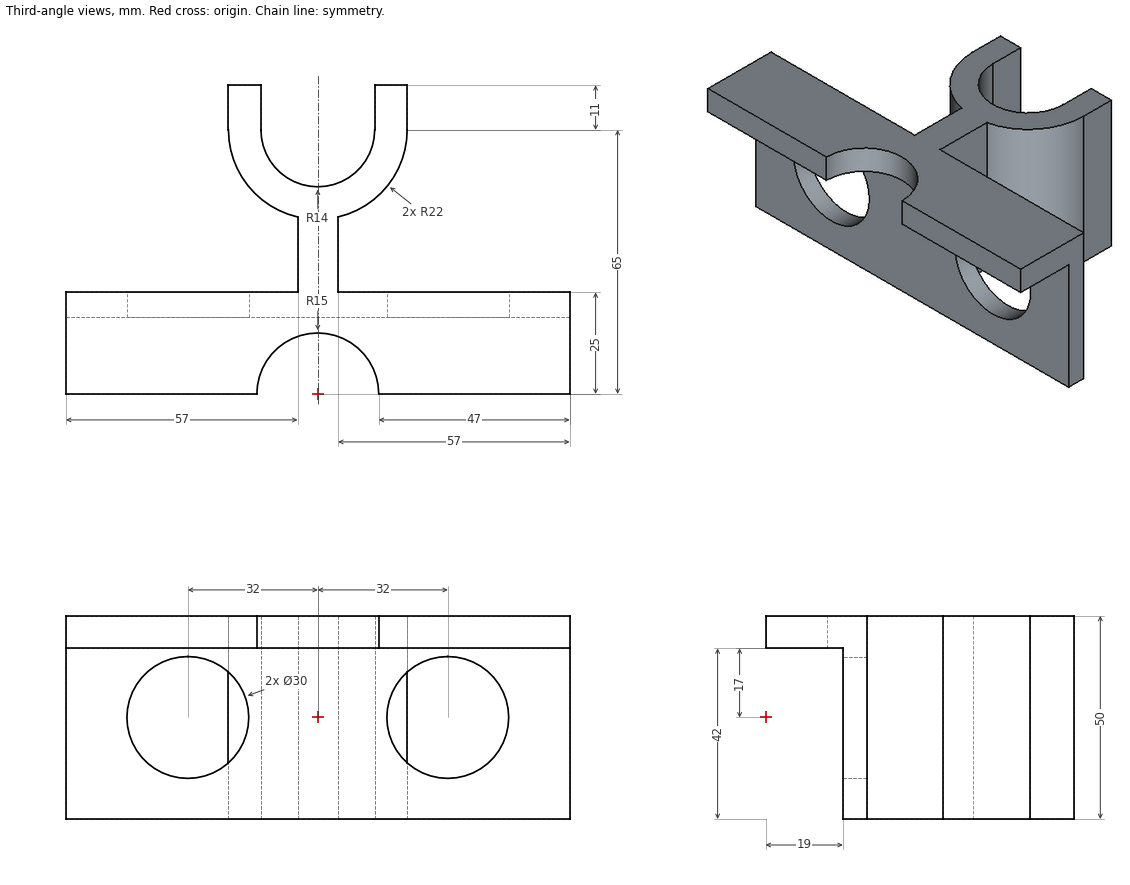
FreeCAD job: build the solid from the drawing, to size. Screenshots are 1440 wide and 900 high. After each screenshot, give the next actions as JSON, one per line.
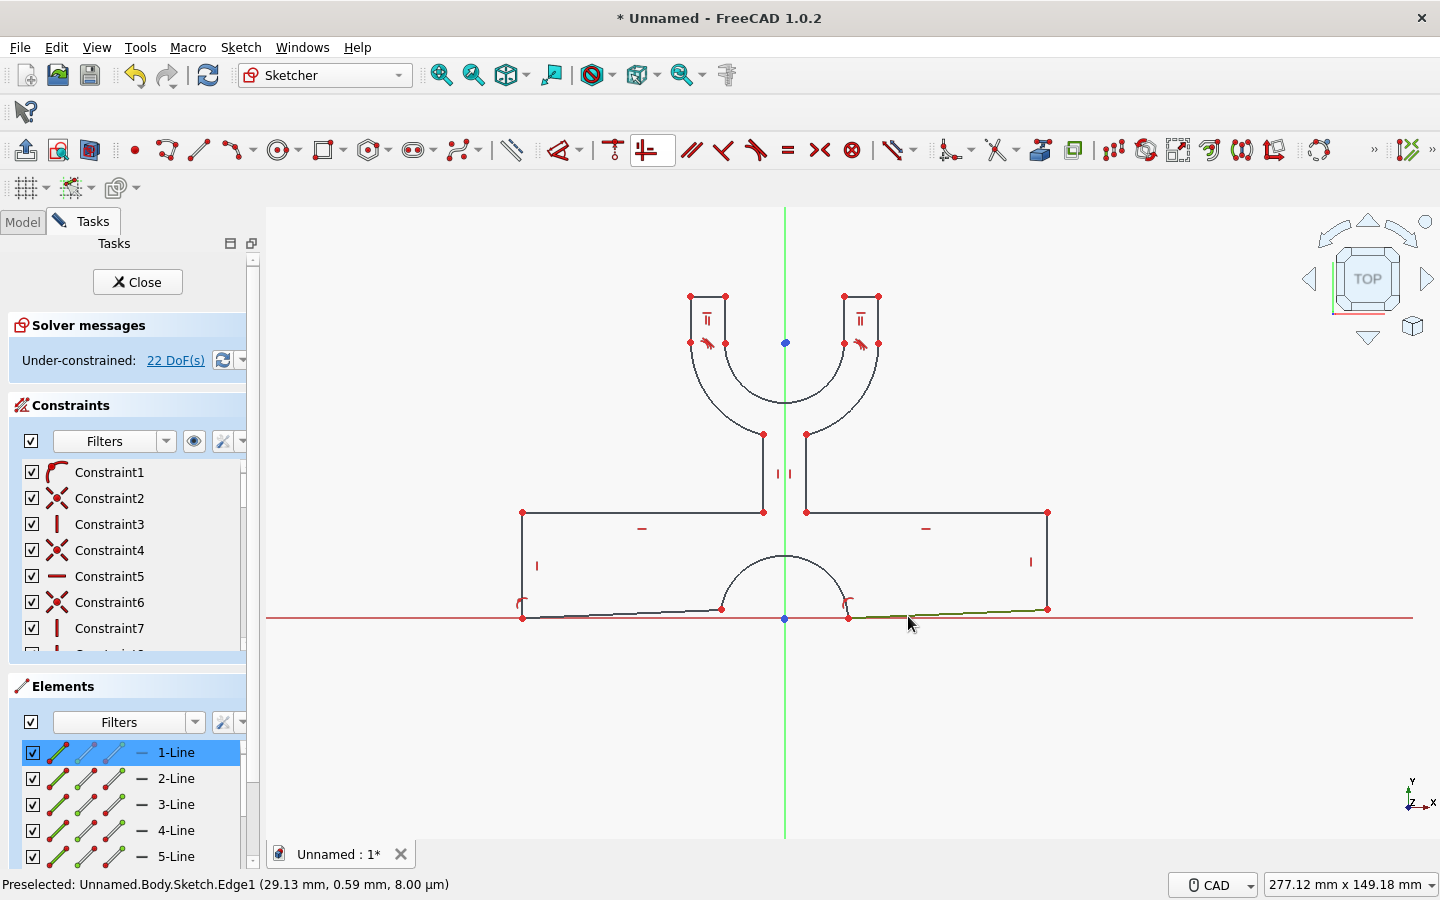
{"action": "key", "text": "h"}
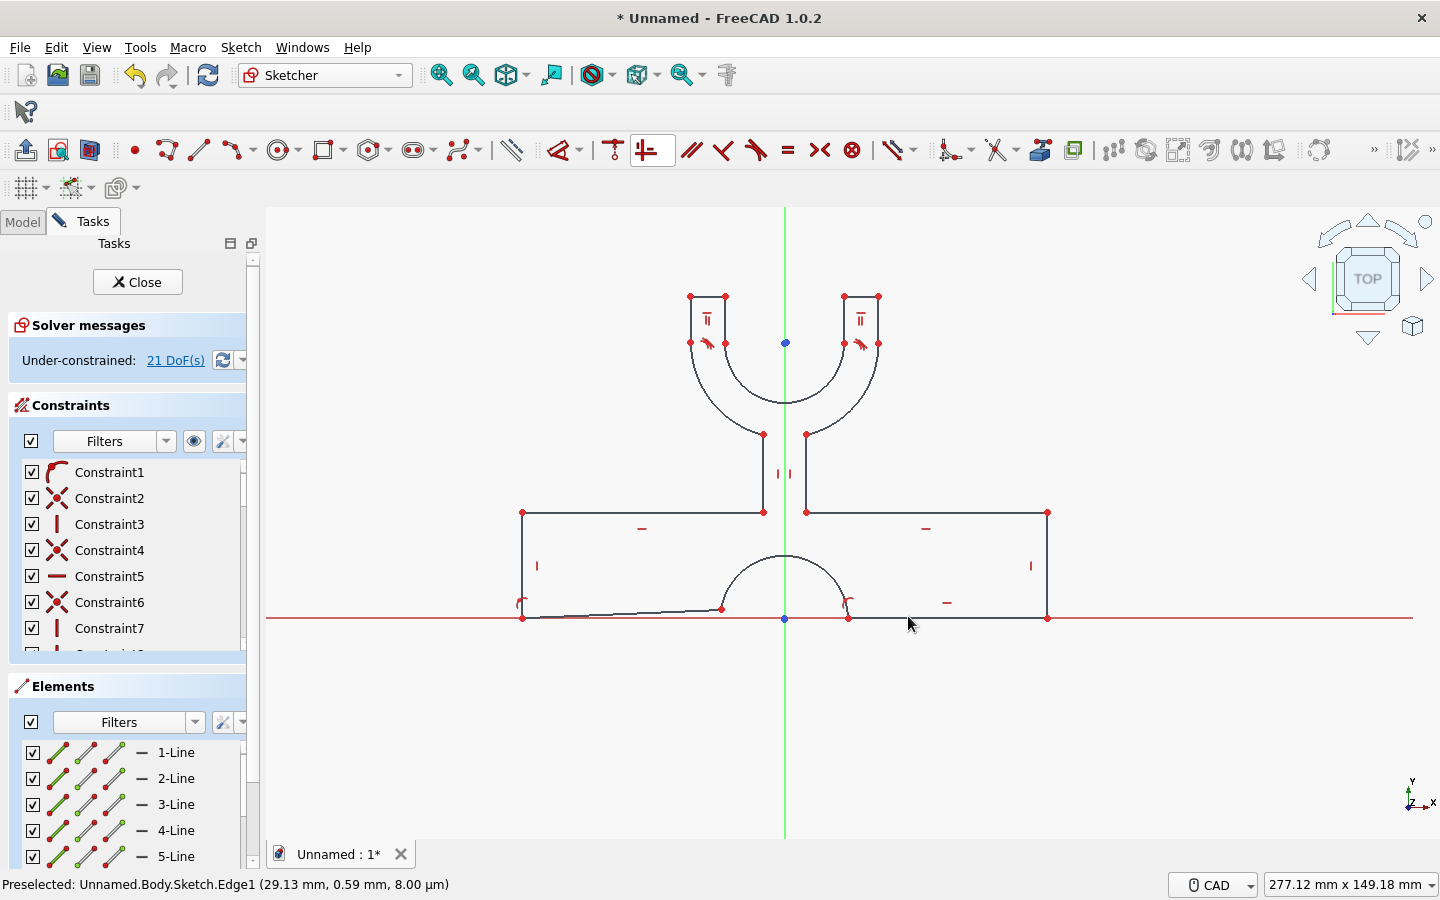
{"action": "left_click", "coordinate": [582, 616]}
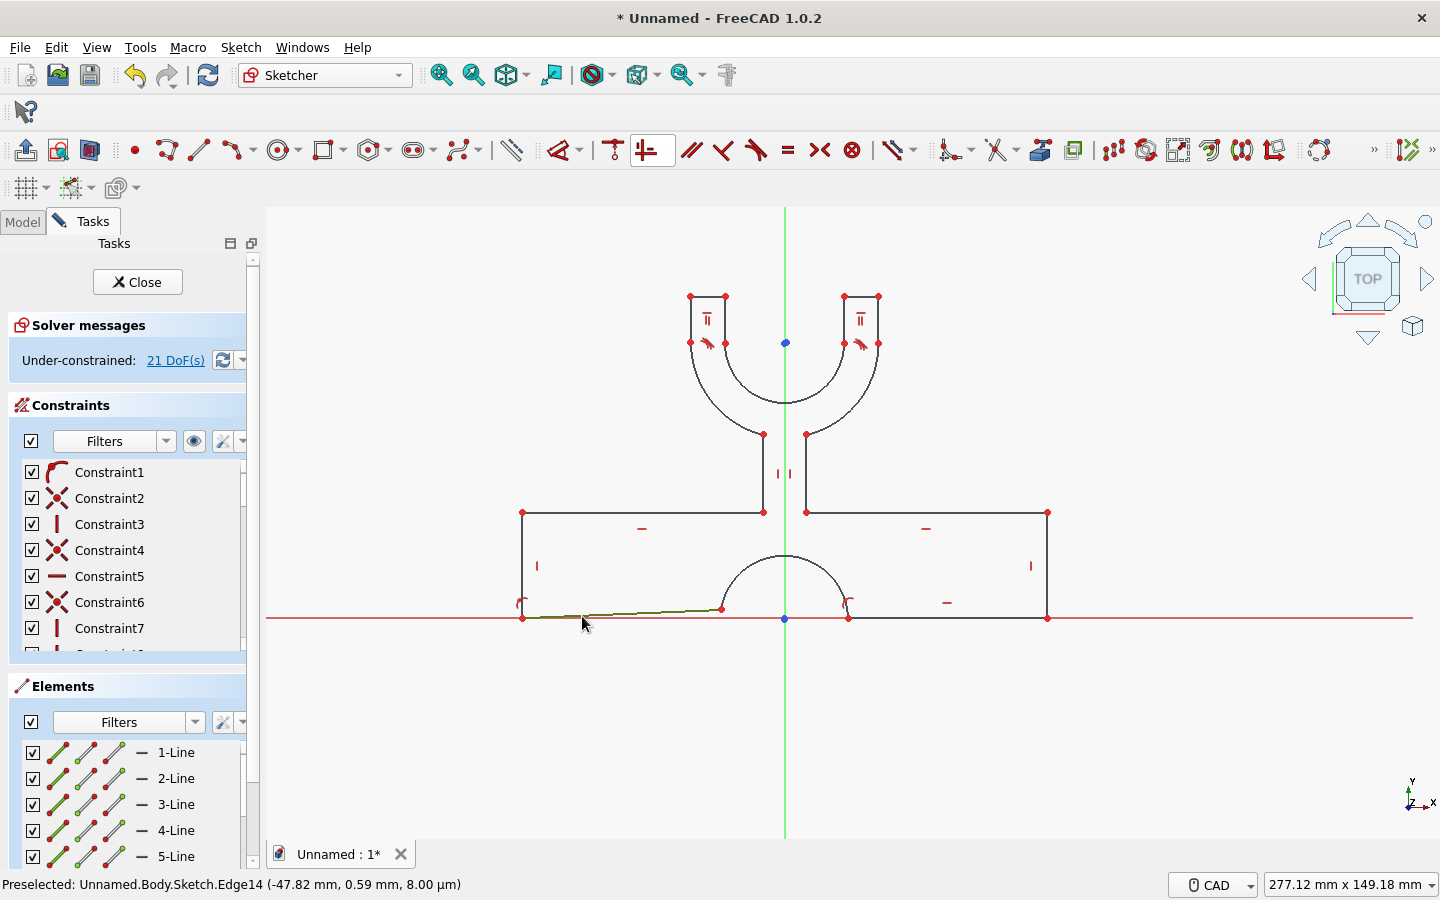
{"action": "left_click", "coordinate": [670, 150]}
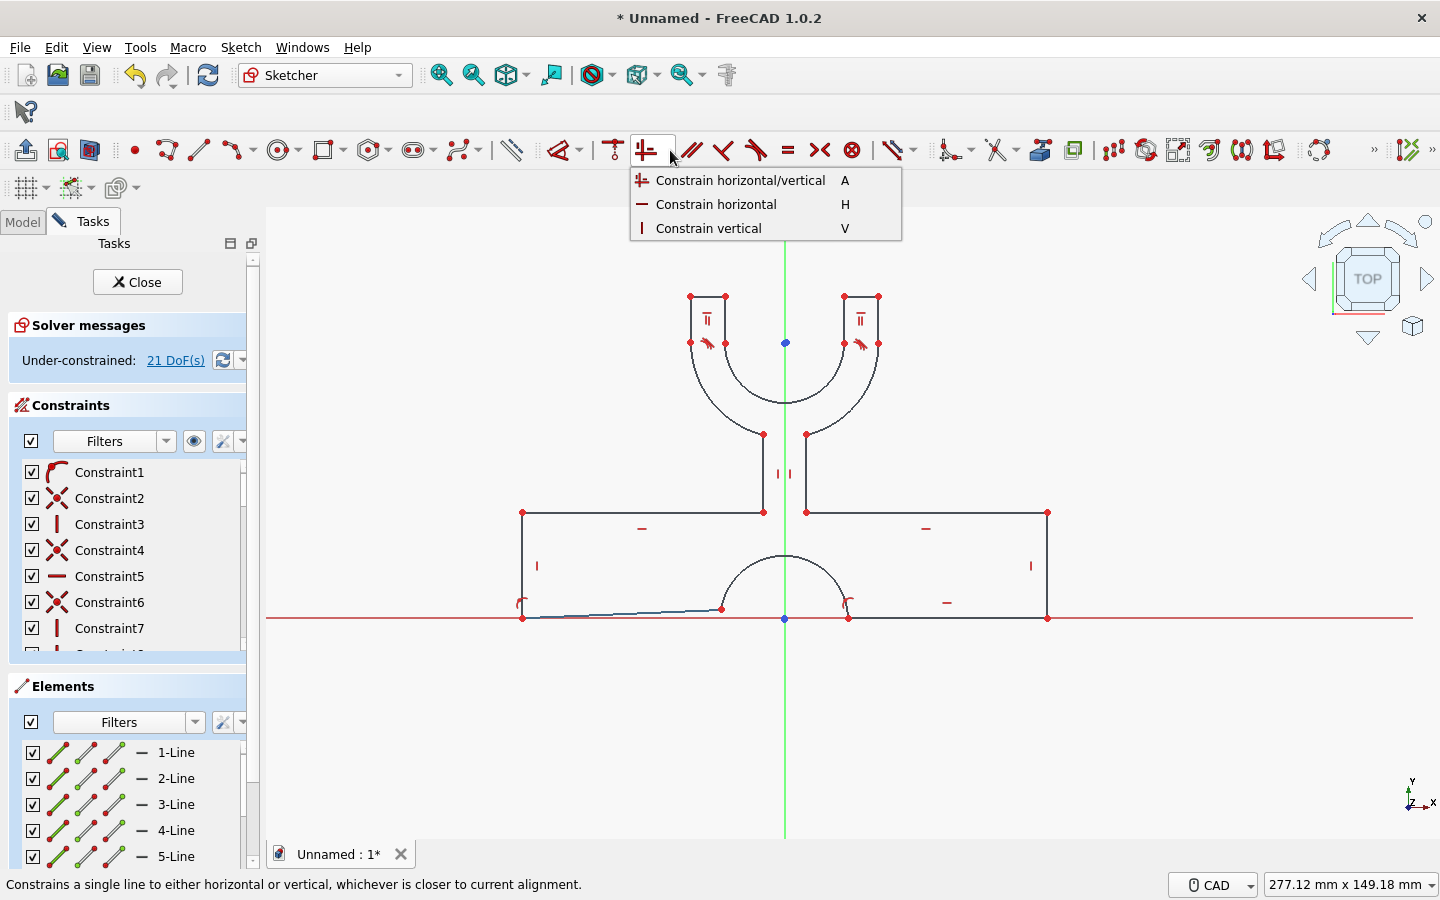
{"action": "left_click", "coordinate": [766, 204]}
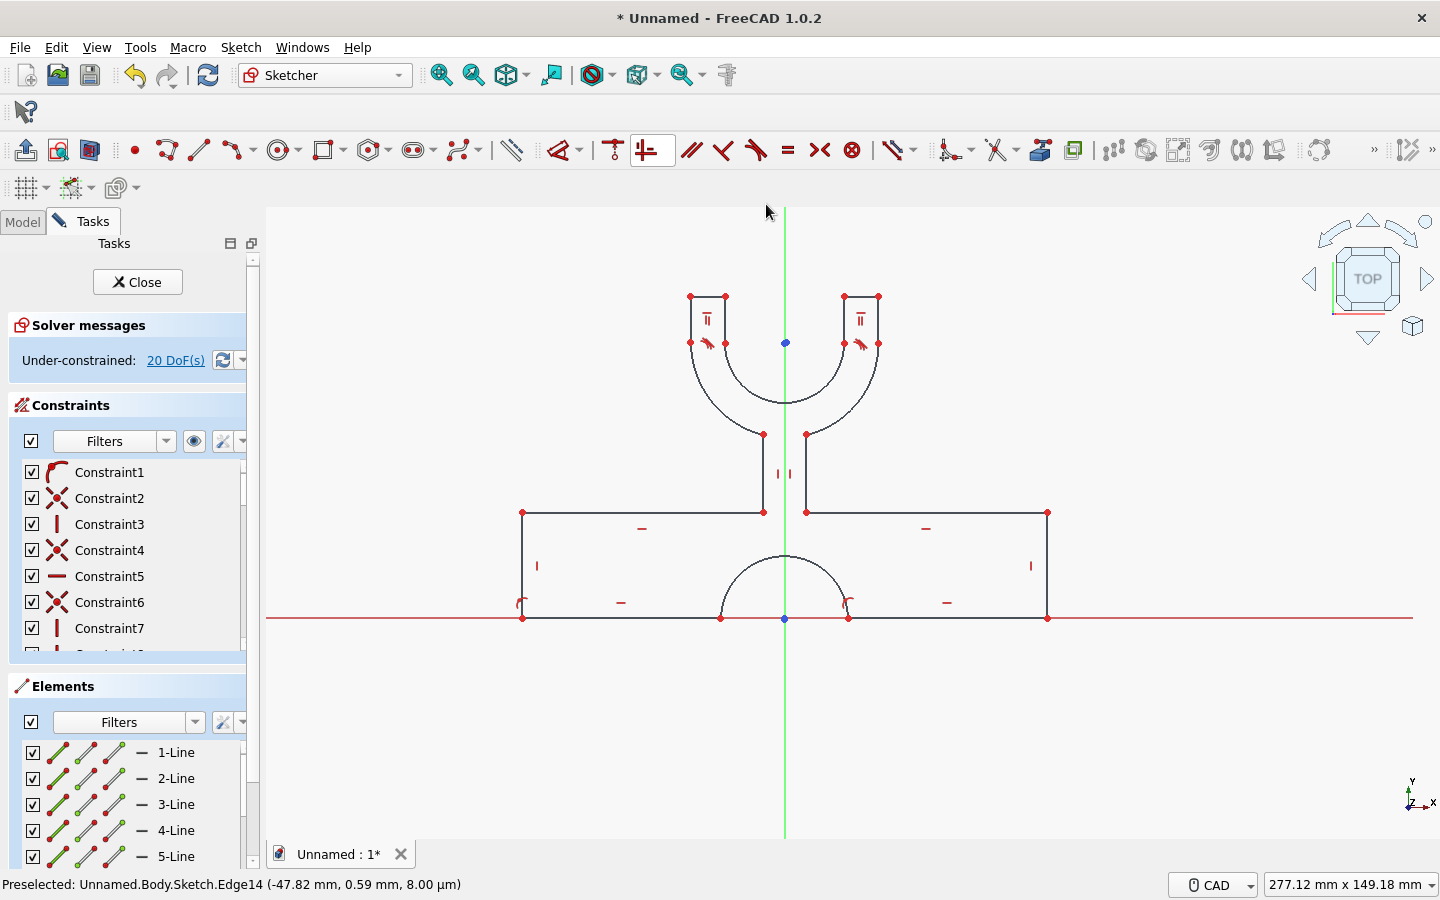
{"action": "left_click", "coordinate": [840, 419]}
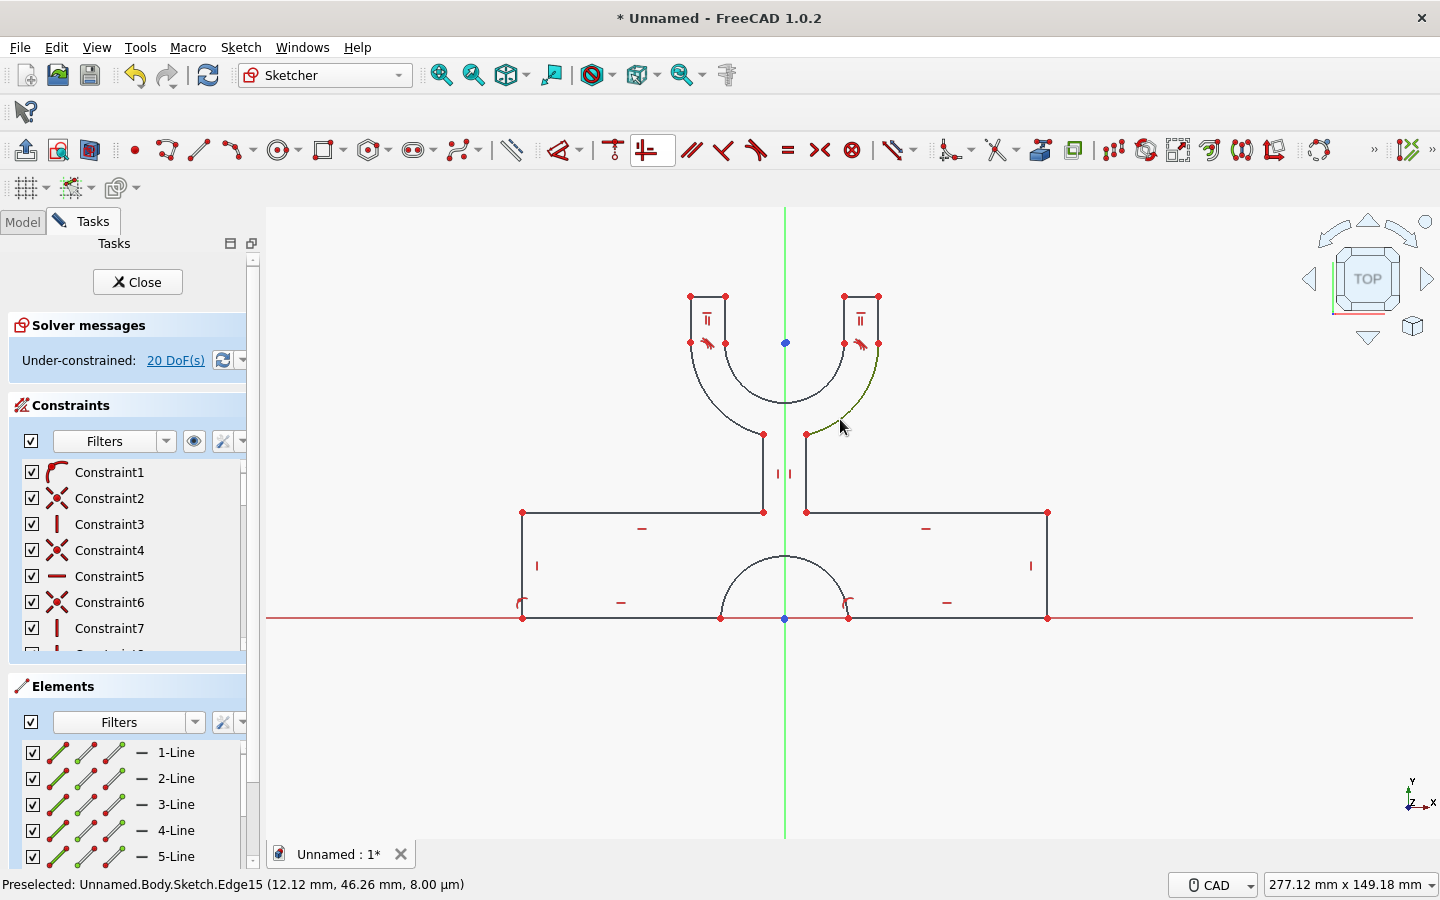
{"action": "left_click", "coordinate": [750, 392]}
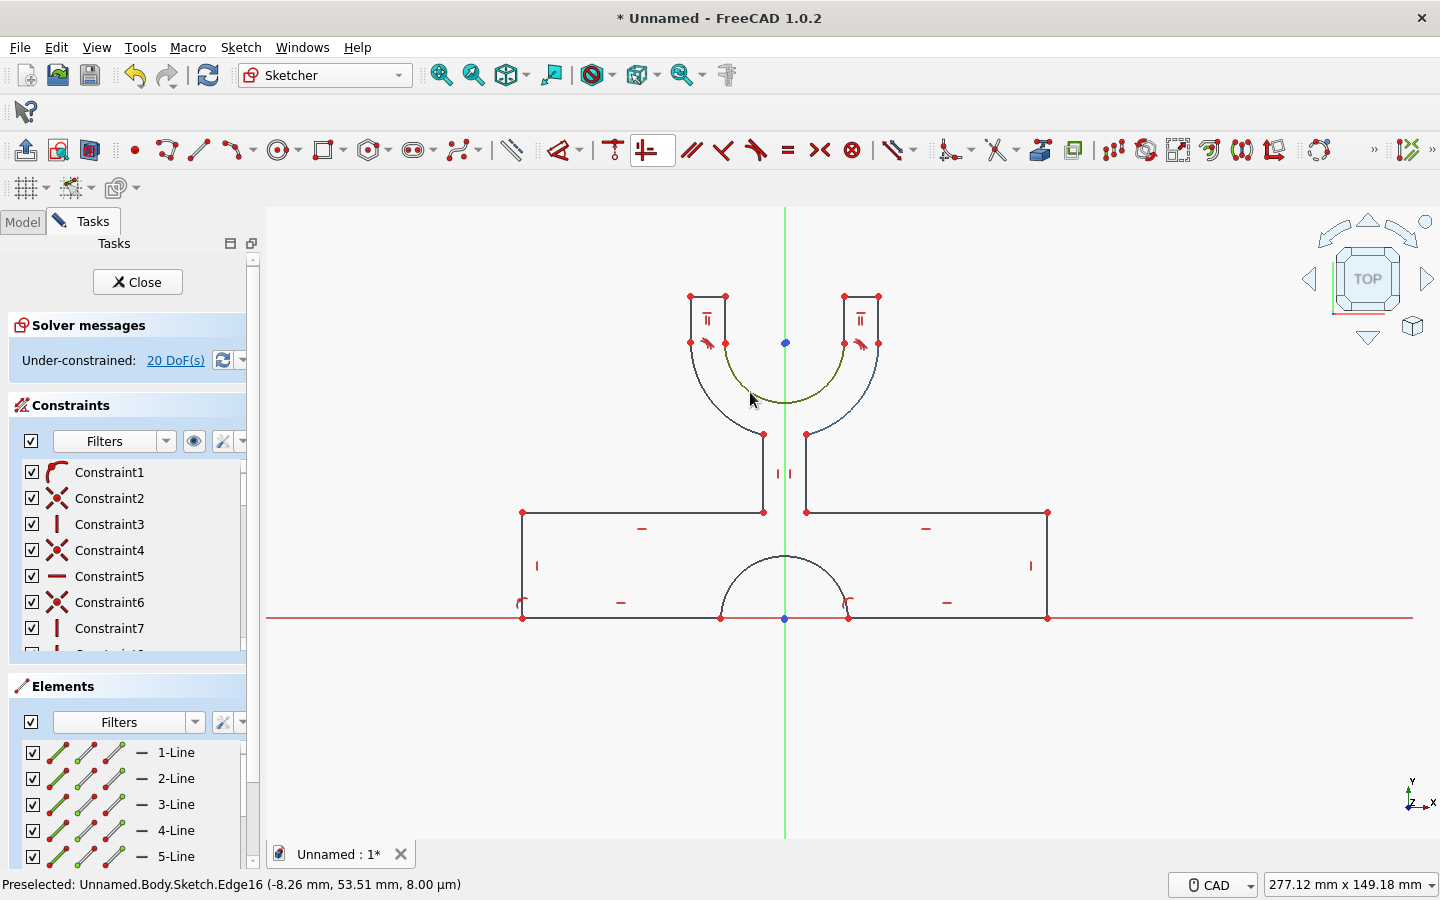
{"action": "left_click", "coordinate": [614, 150]}